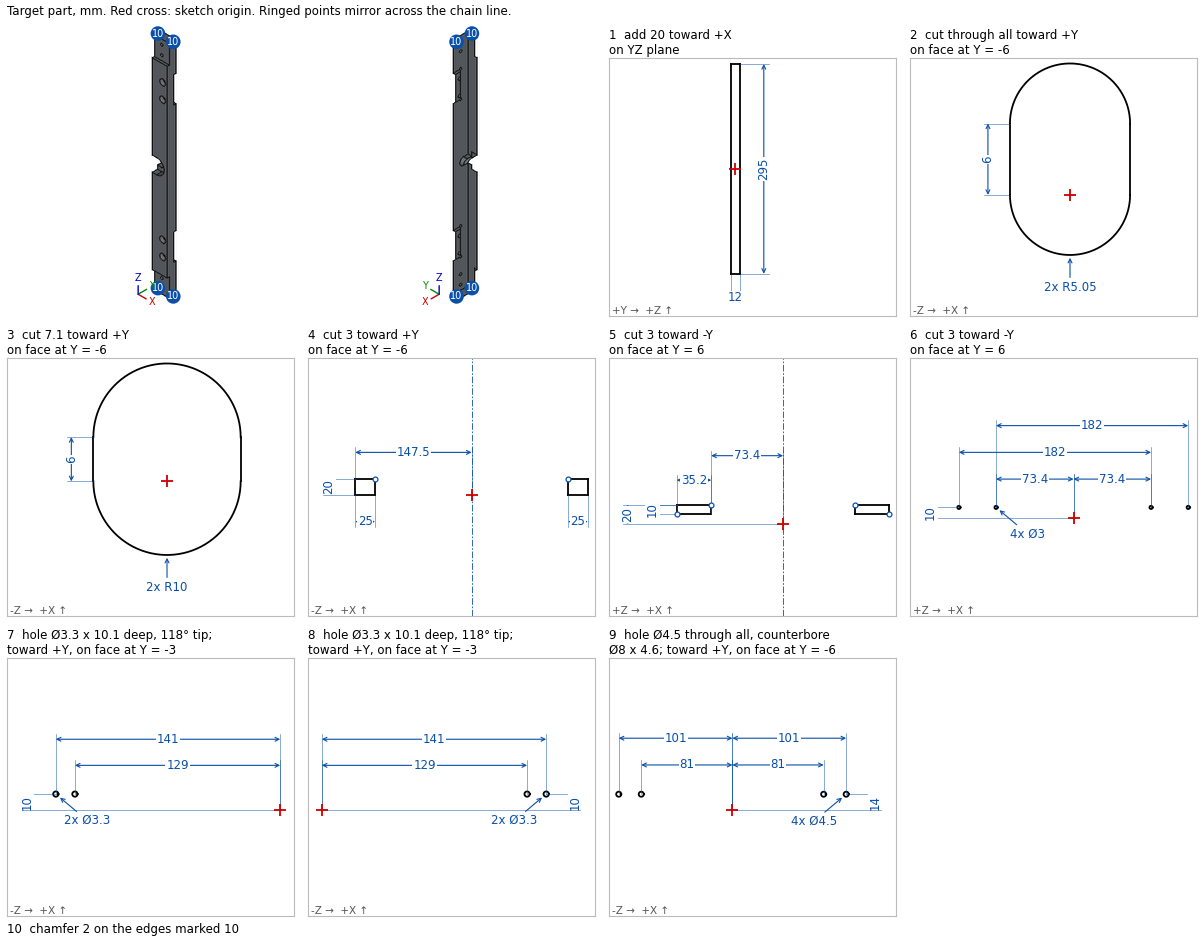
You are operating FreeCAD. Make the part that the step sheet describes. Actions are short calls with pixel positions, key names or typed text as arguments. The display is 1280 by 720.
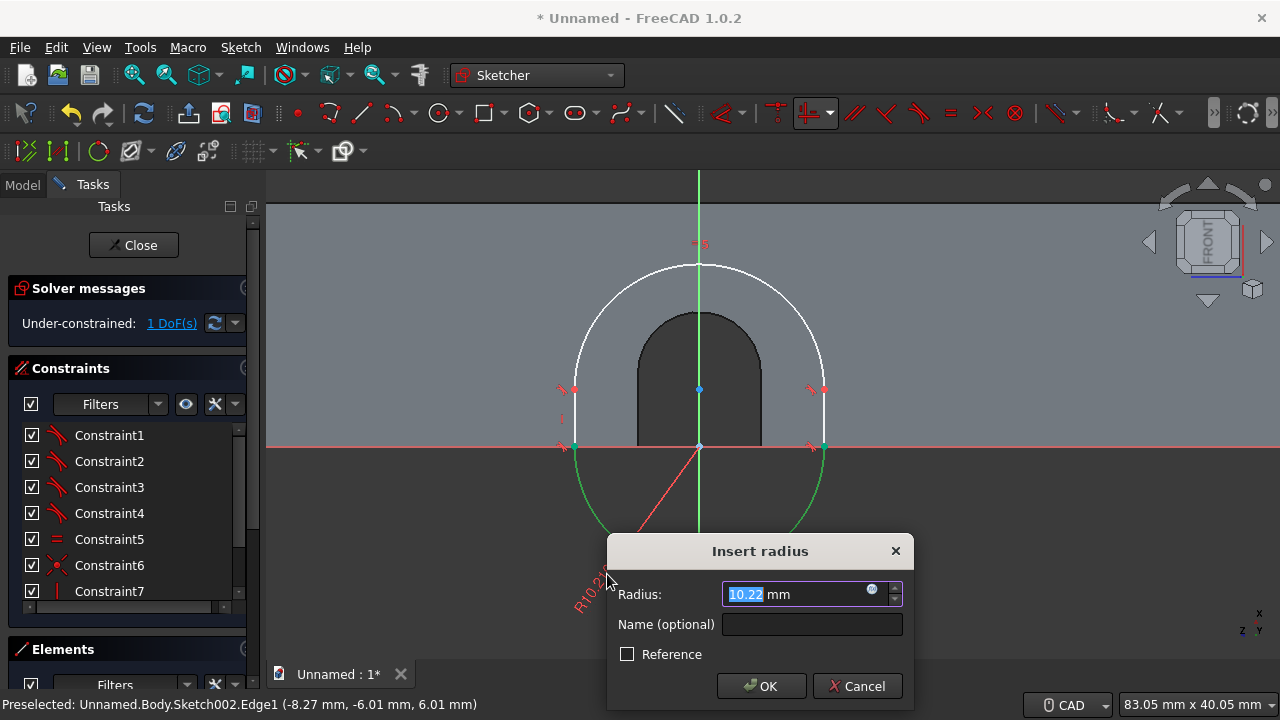
text(10)
key(Return)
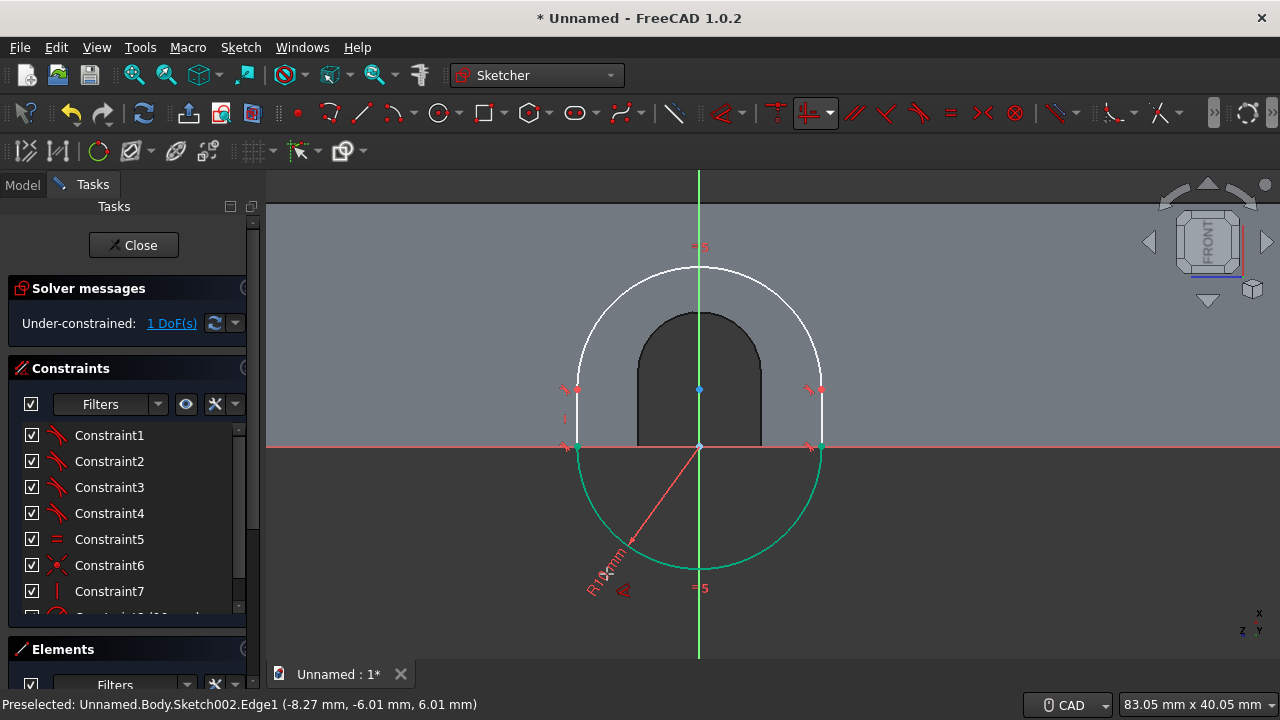
click(577, 430)
click(543, 418)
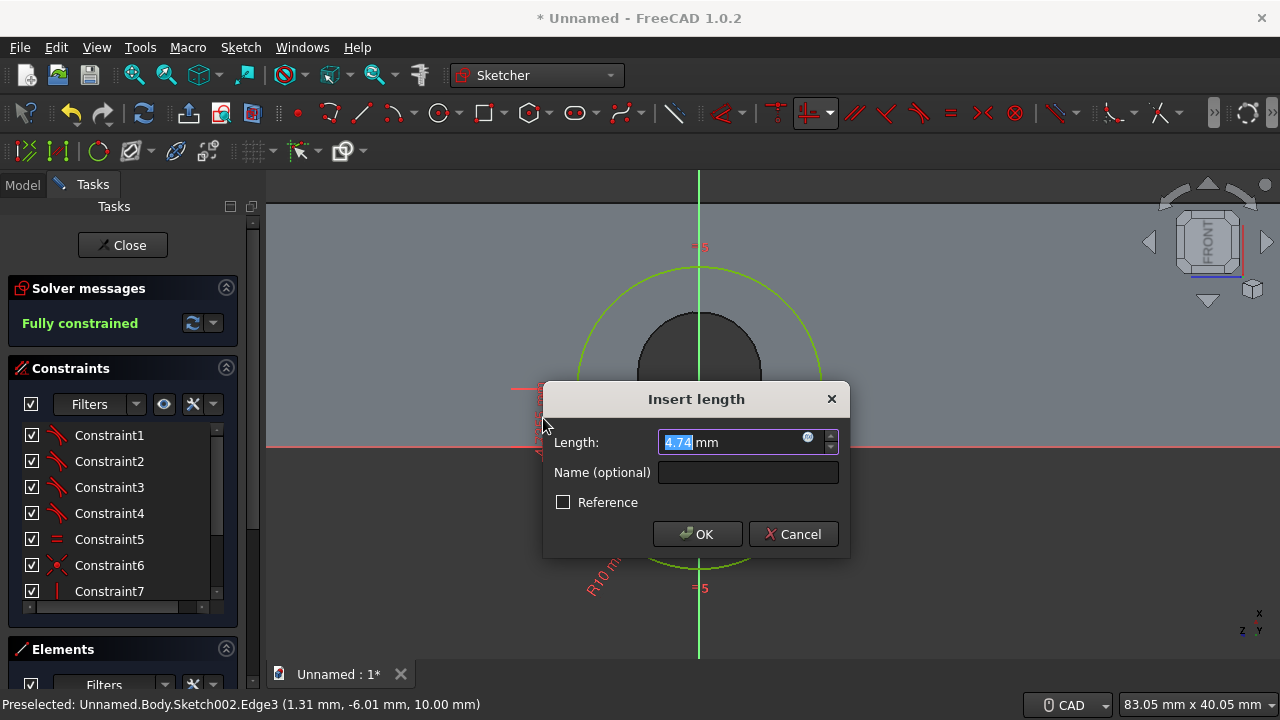
text(6)
key(Return)
key(Escape)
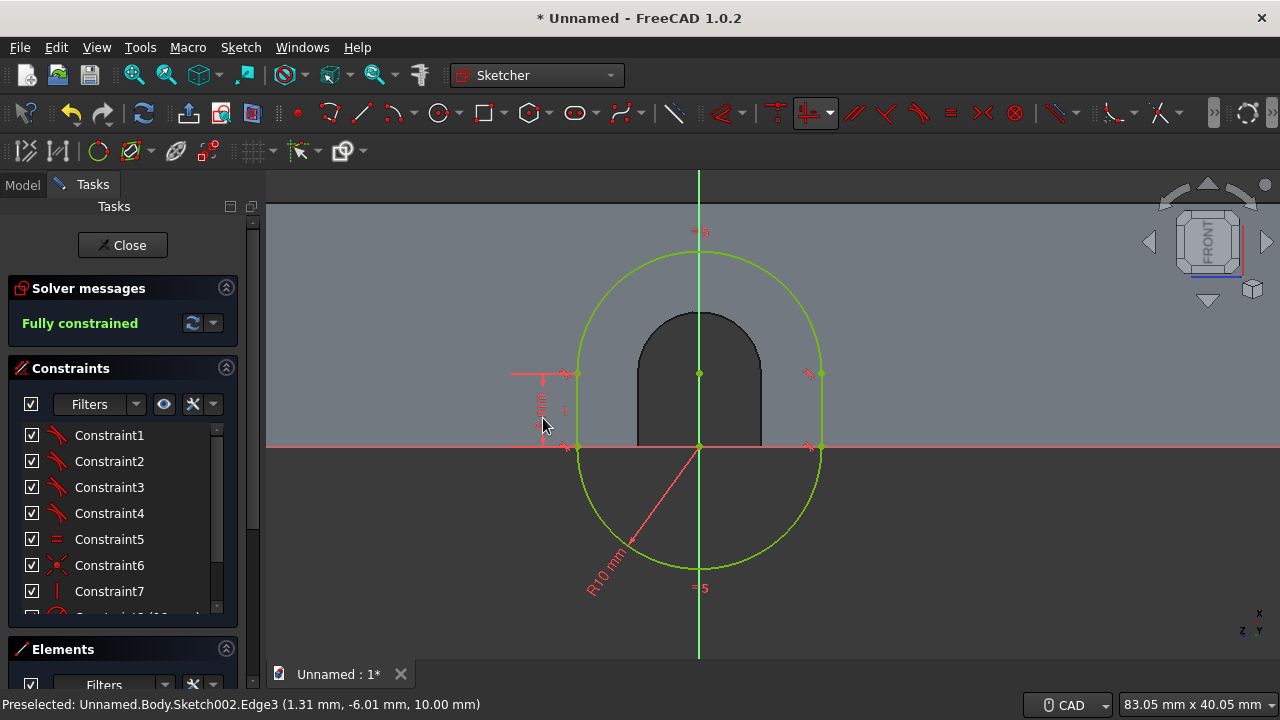
click(123, 245)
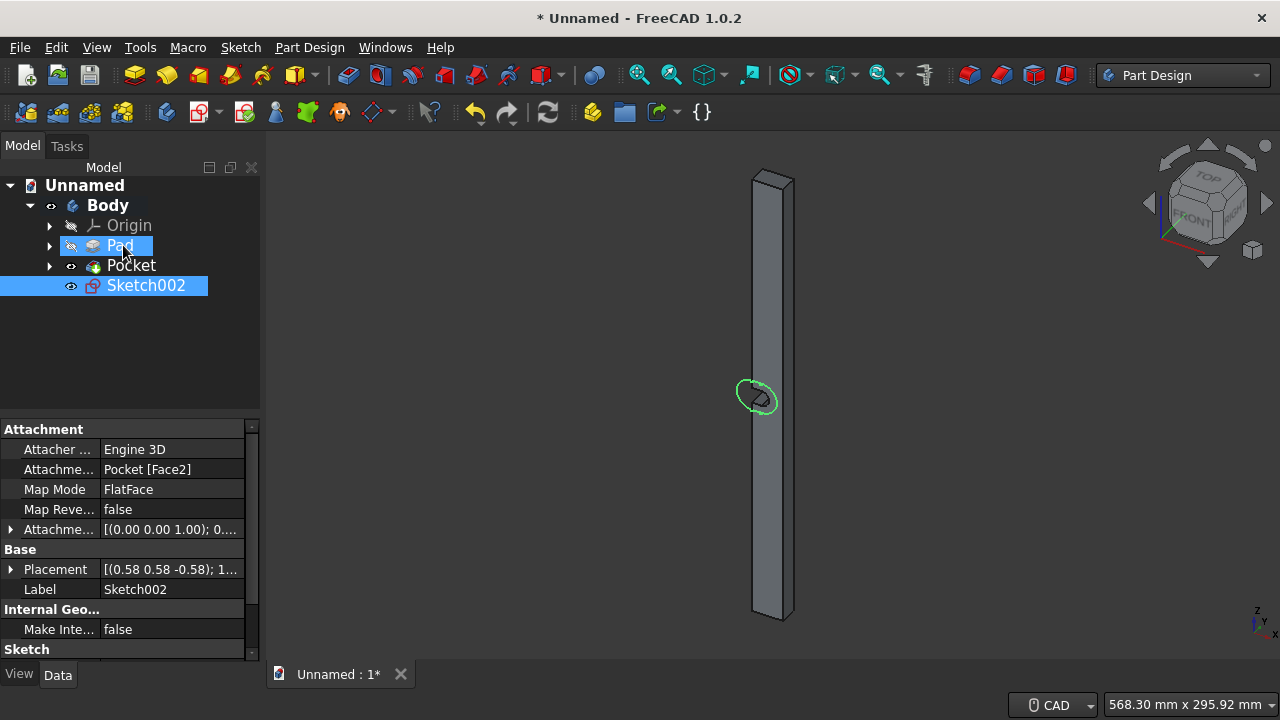
click(350, 76)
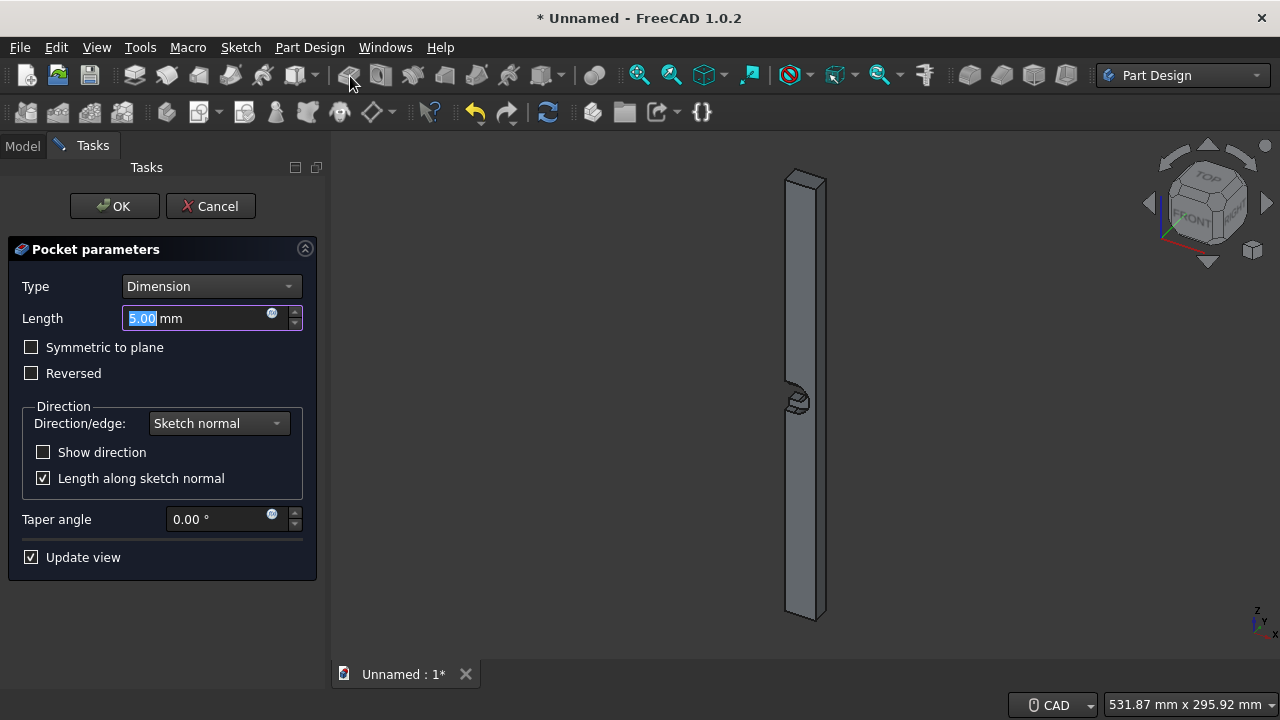
text(7.1)
key(Tab)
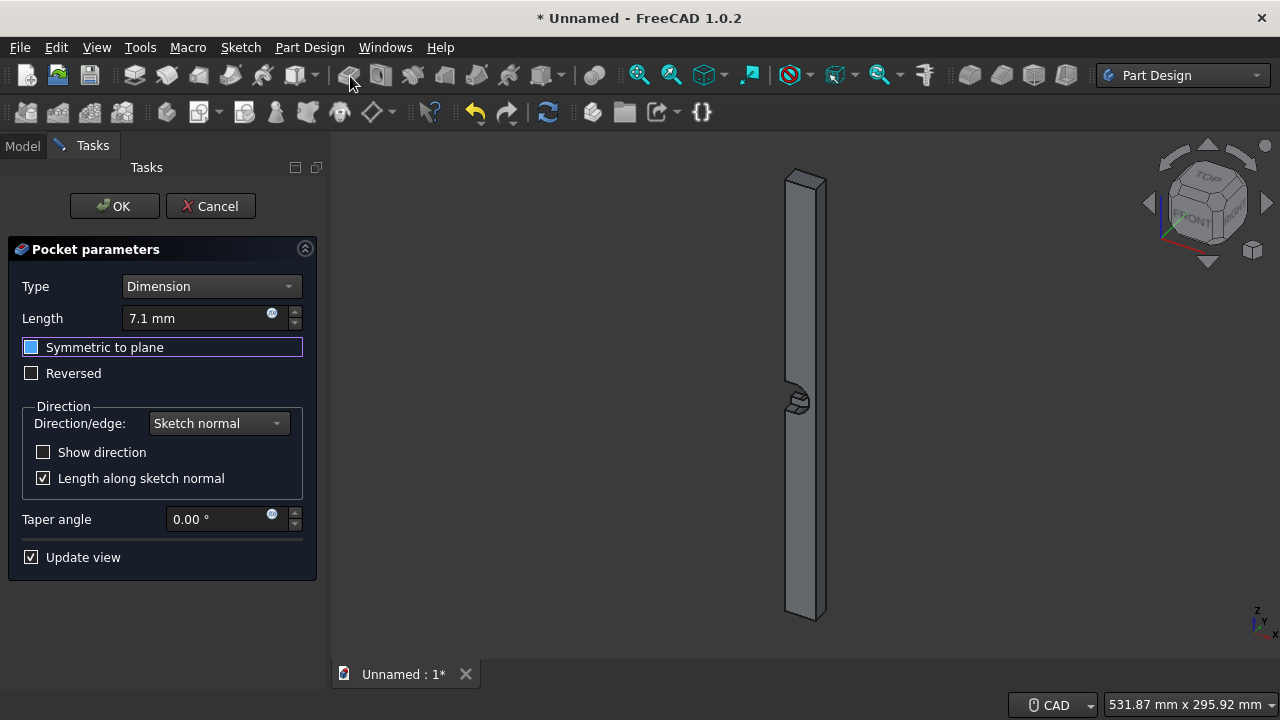
click(115, 206)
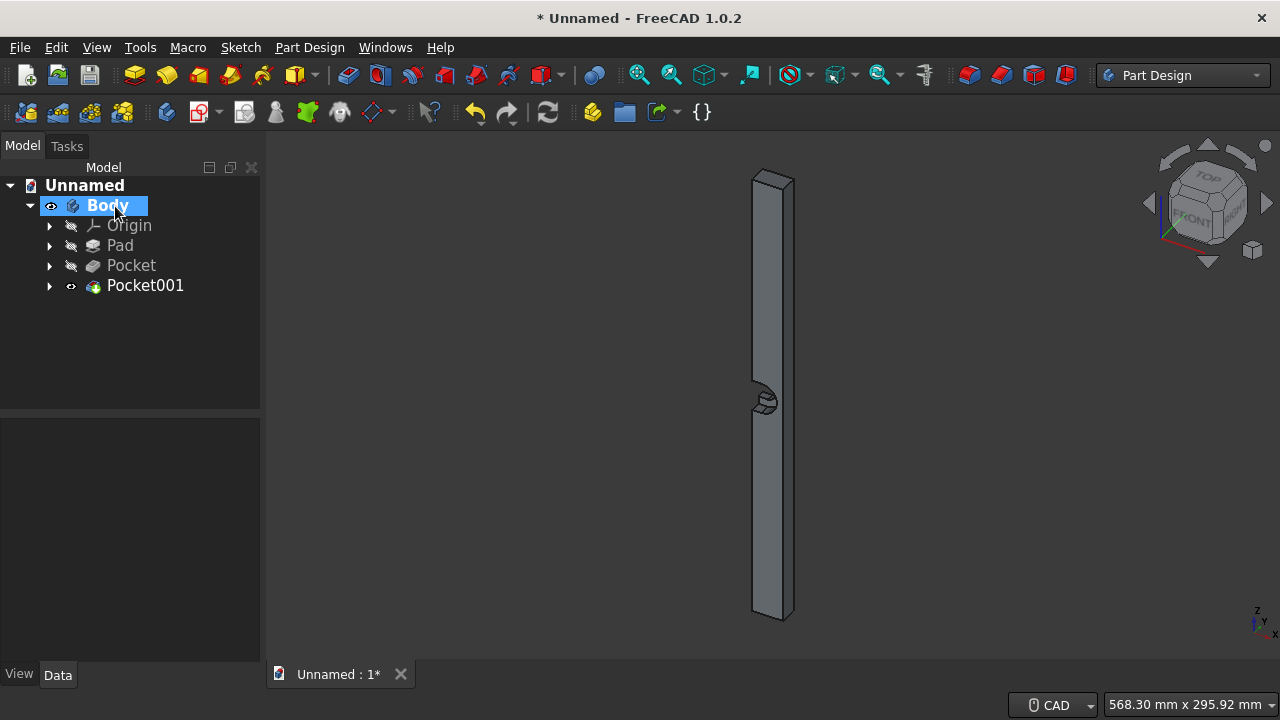
click(768, 523)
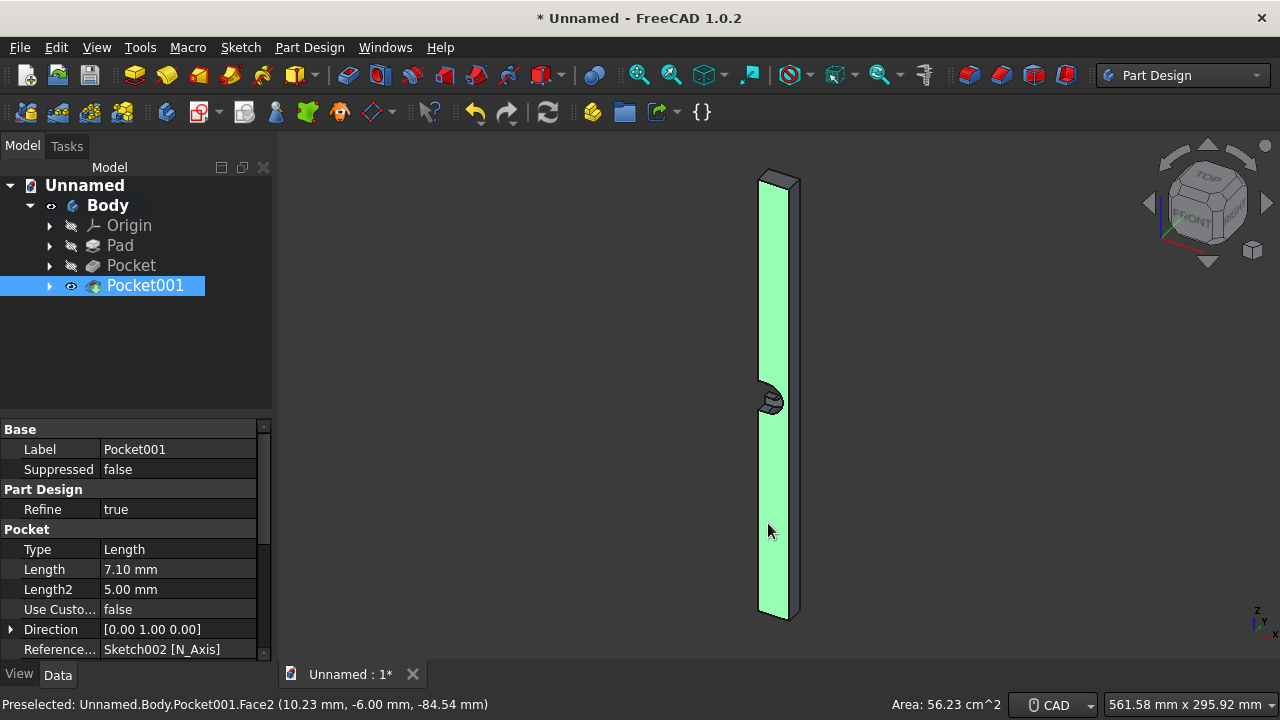
click(200, 112)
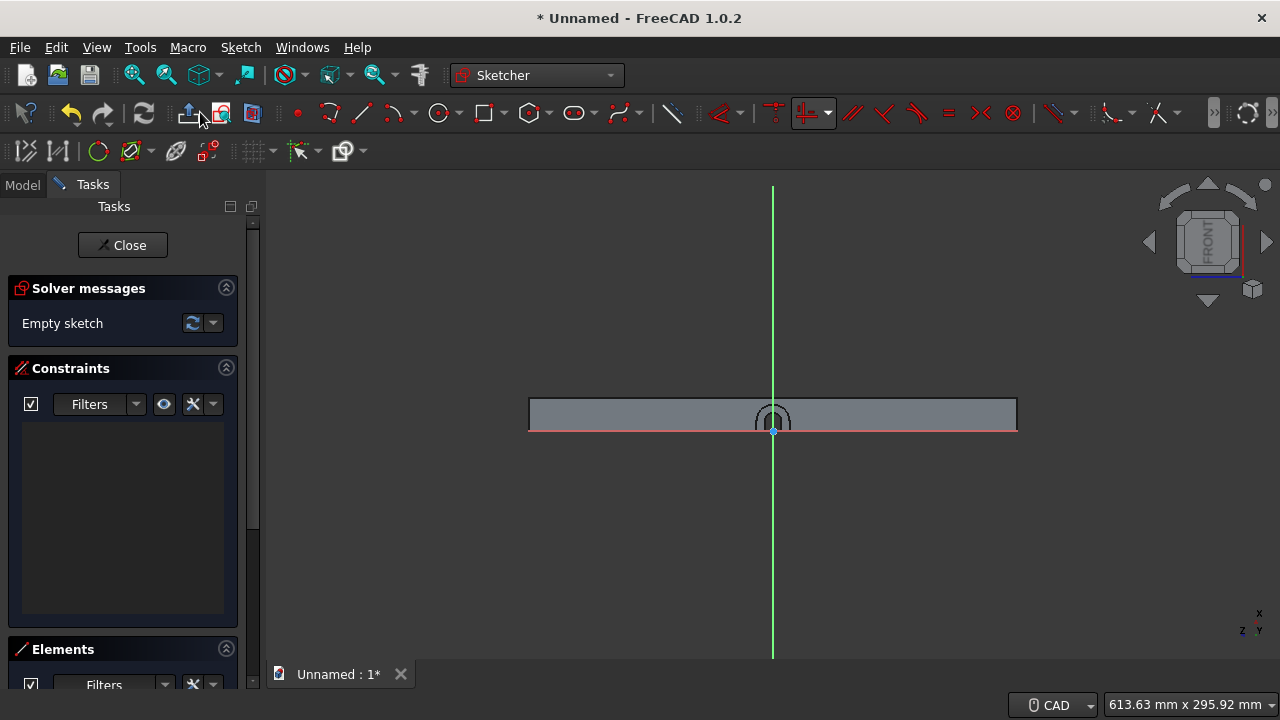
click(484, 114)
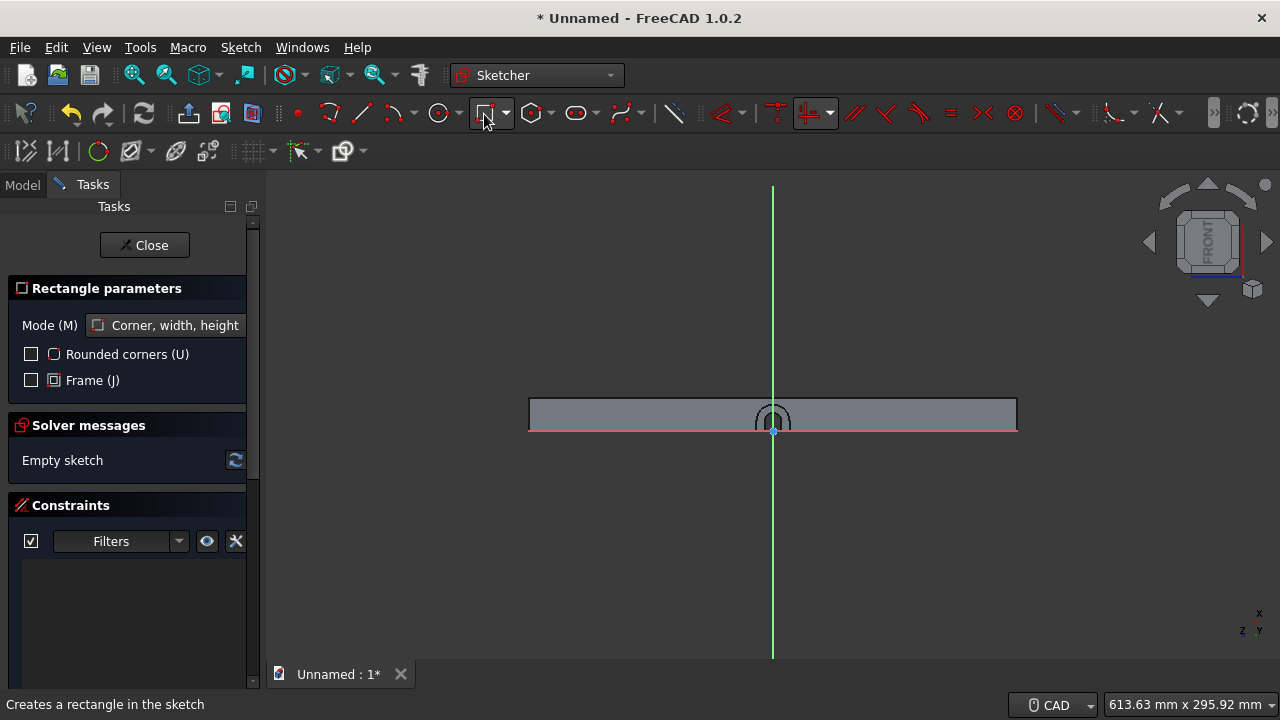
click(529, 398)
click(571, 431)